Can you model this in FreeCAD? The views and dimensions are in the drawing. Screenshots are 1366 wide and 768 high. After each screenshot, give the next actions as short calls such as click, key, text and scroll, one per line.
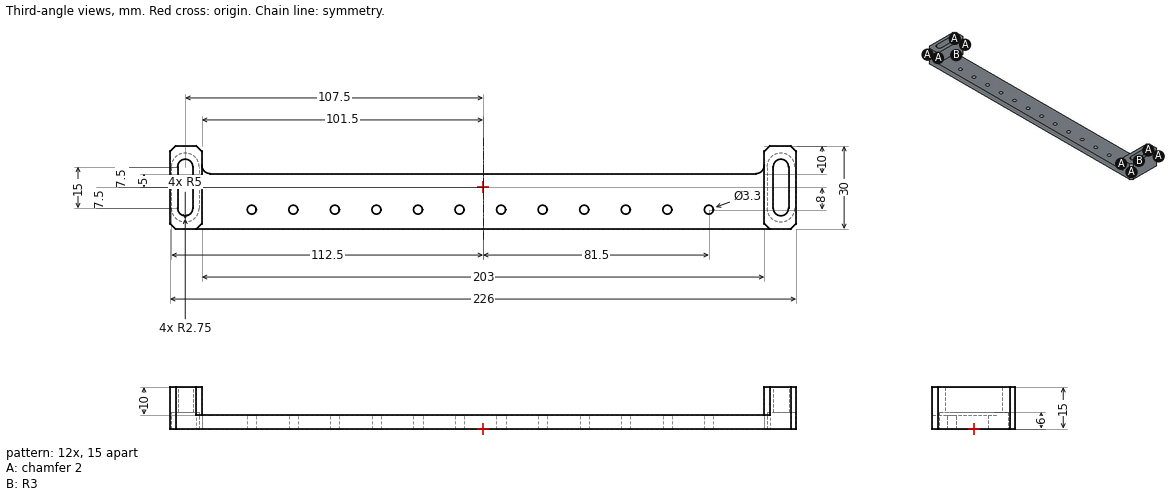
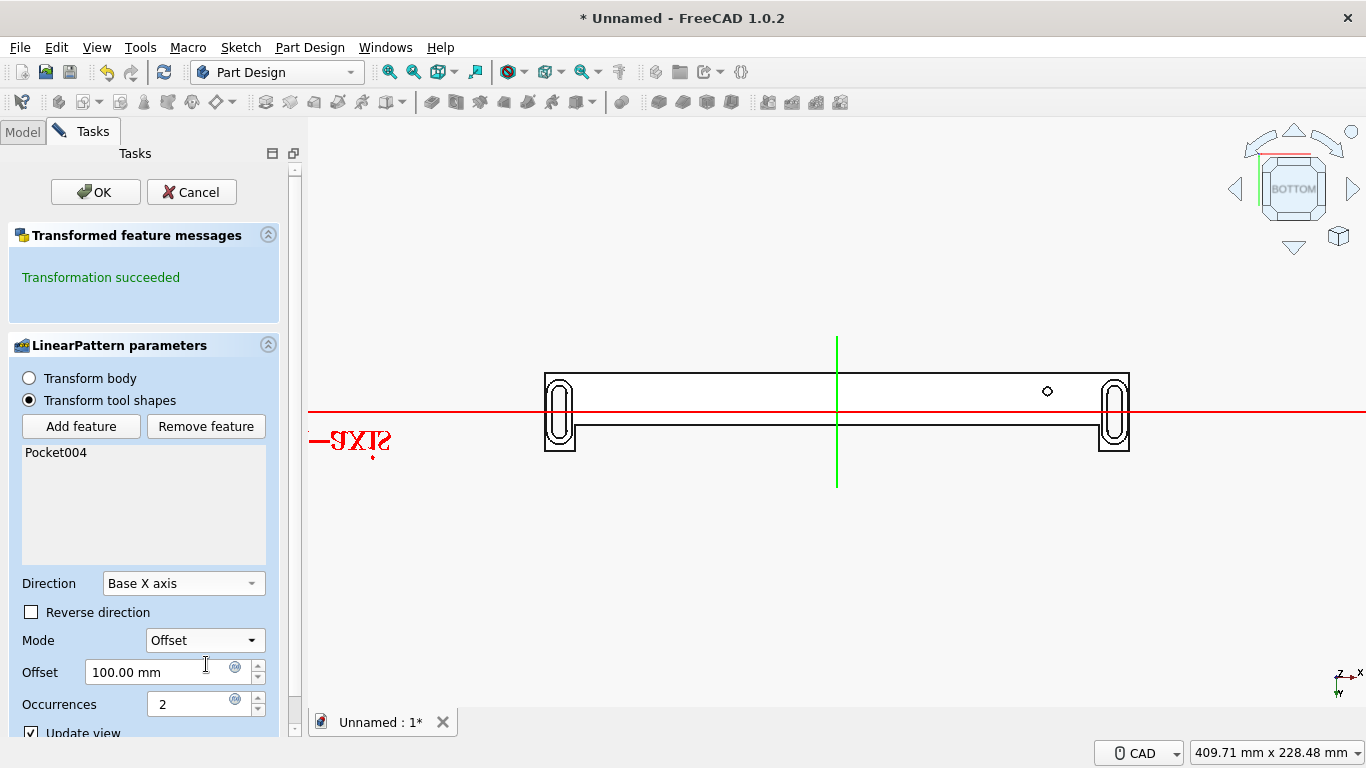
triple_click(168, 672)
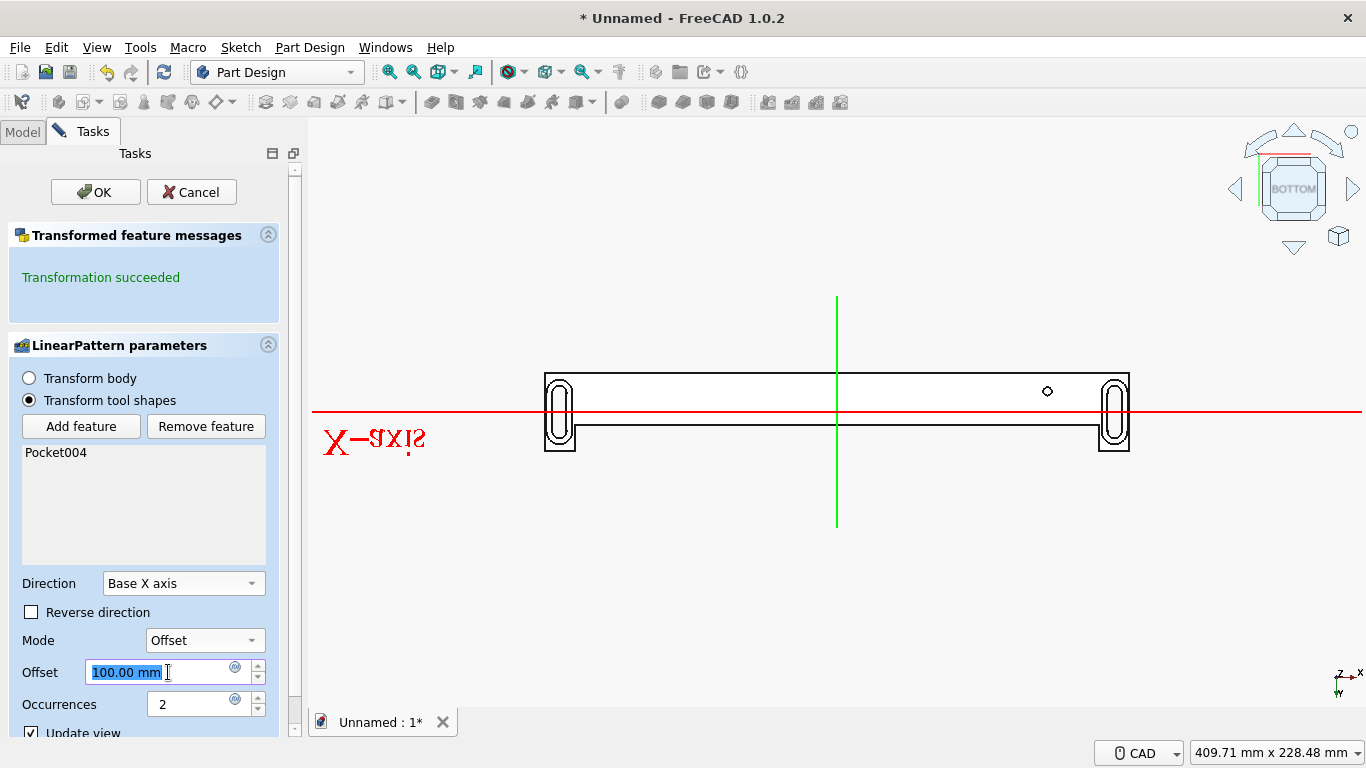
text(15)
key(Tab)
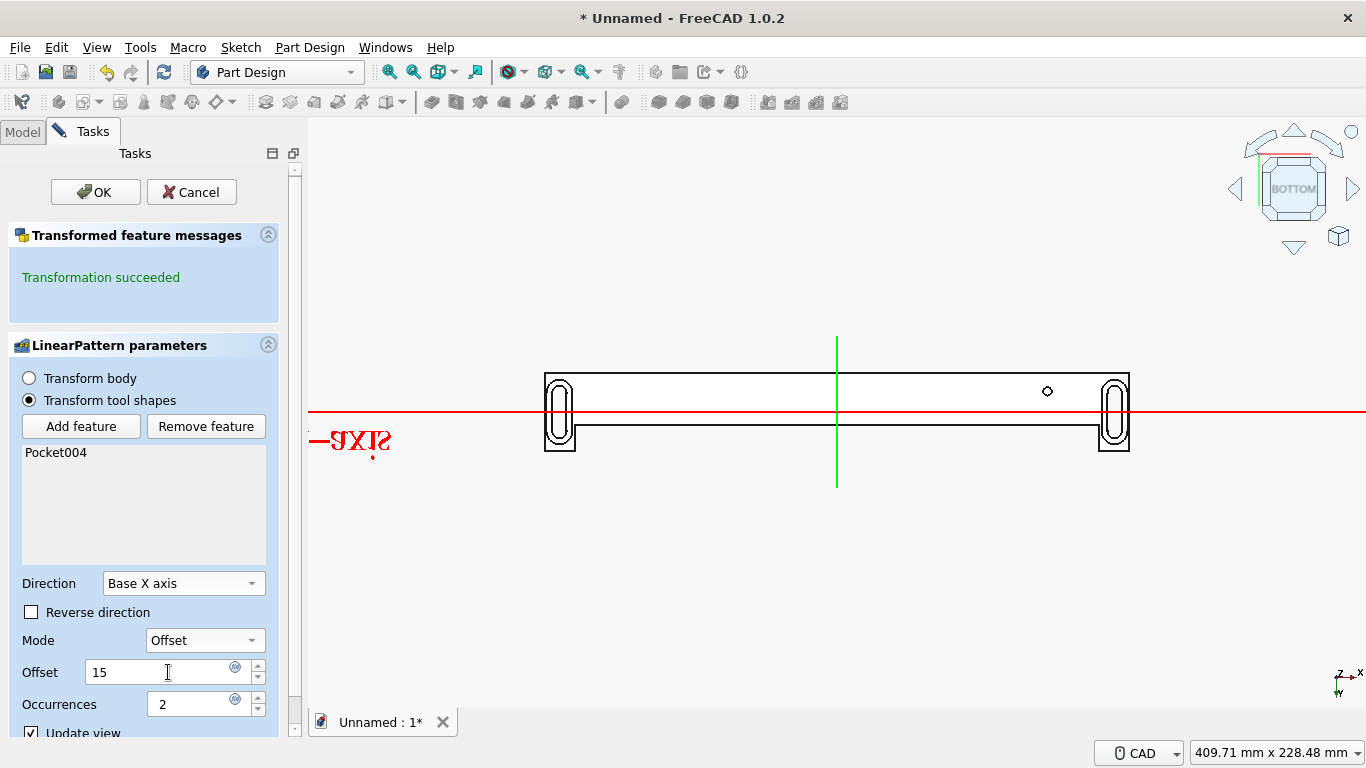
triple_click(198, 704)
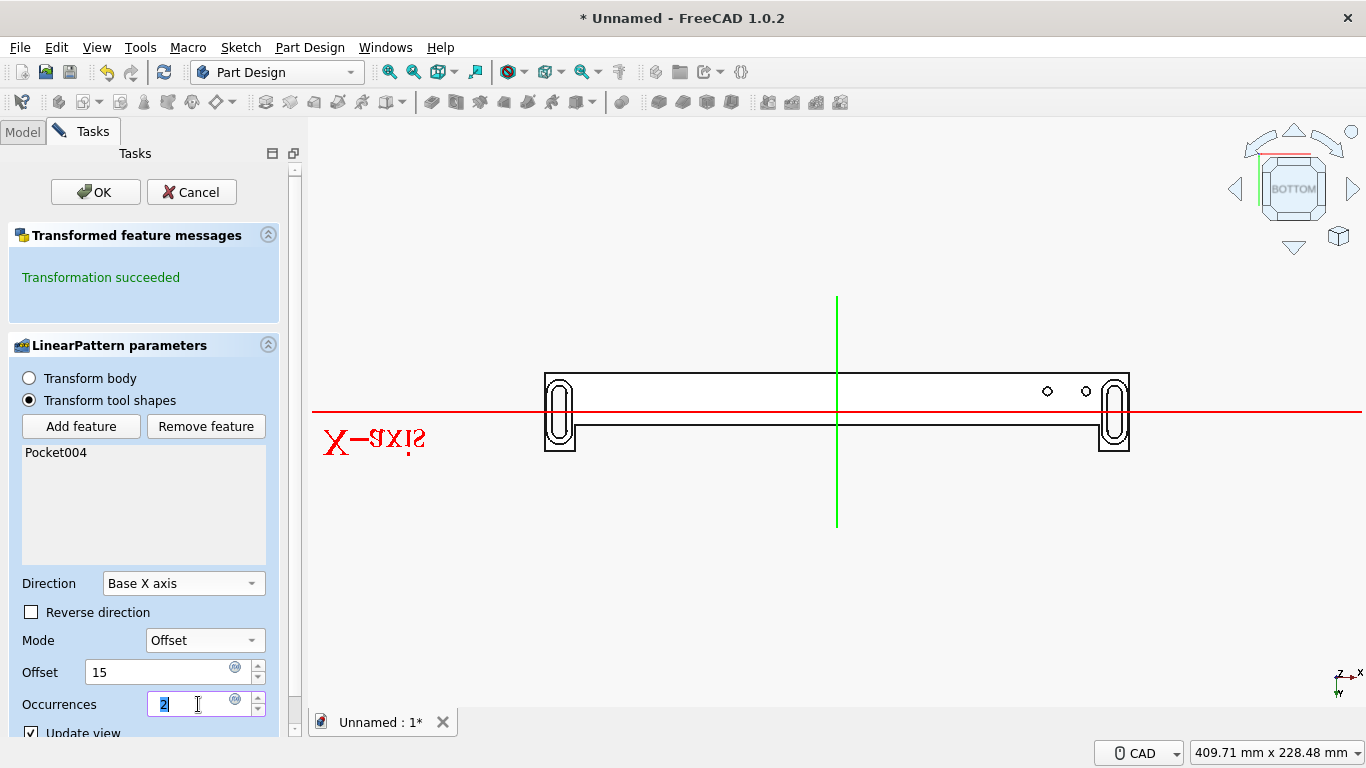
text(12)
key(Tab)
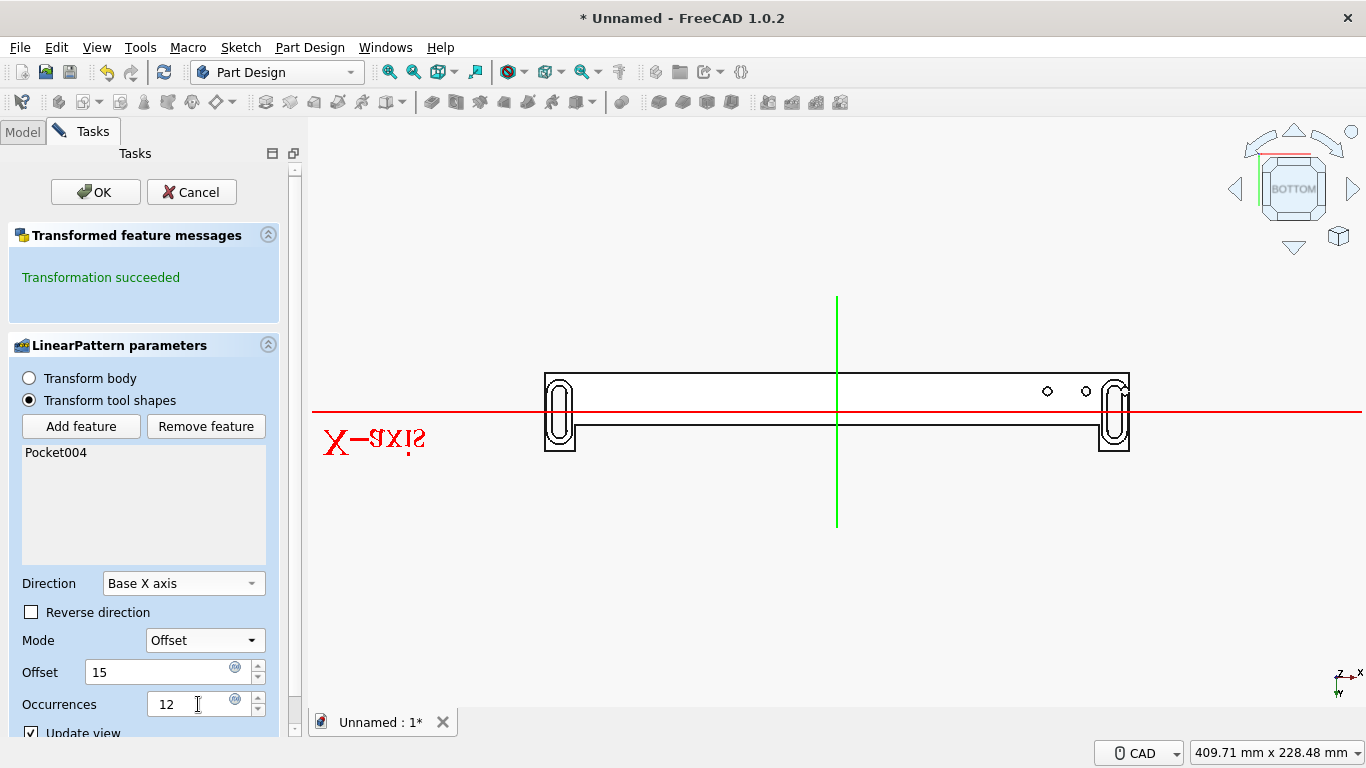
click(30, 612)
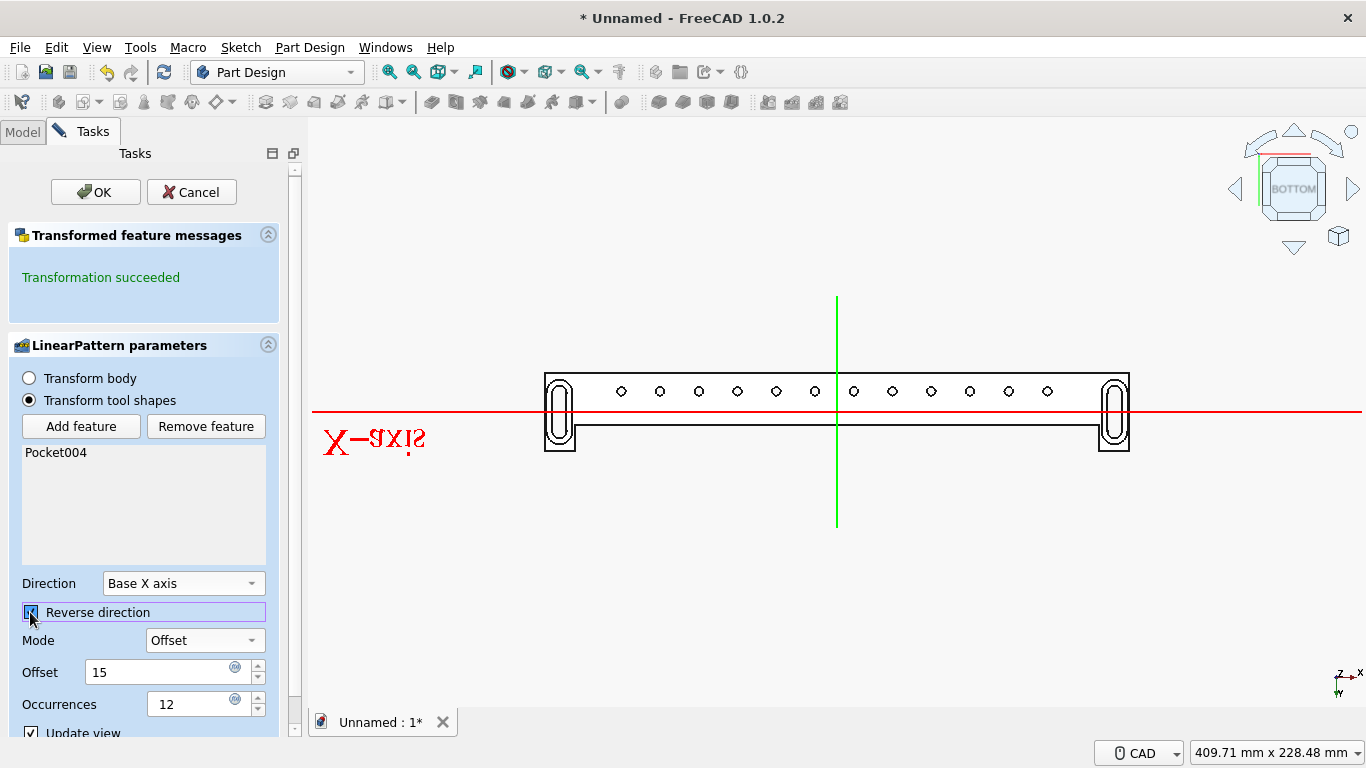
click(96, 192)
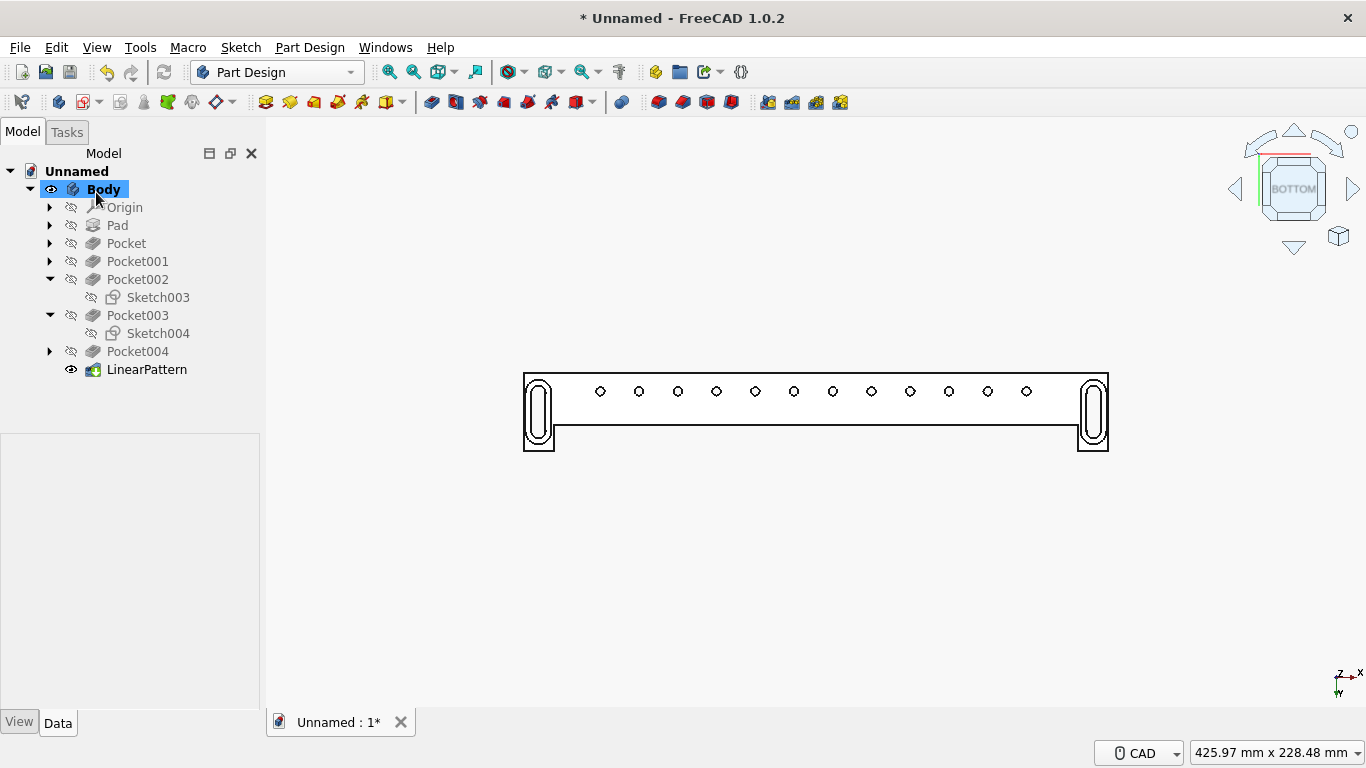
key(0)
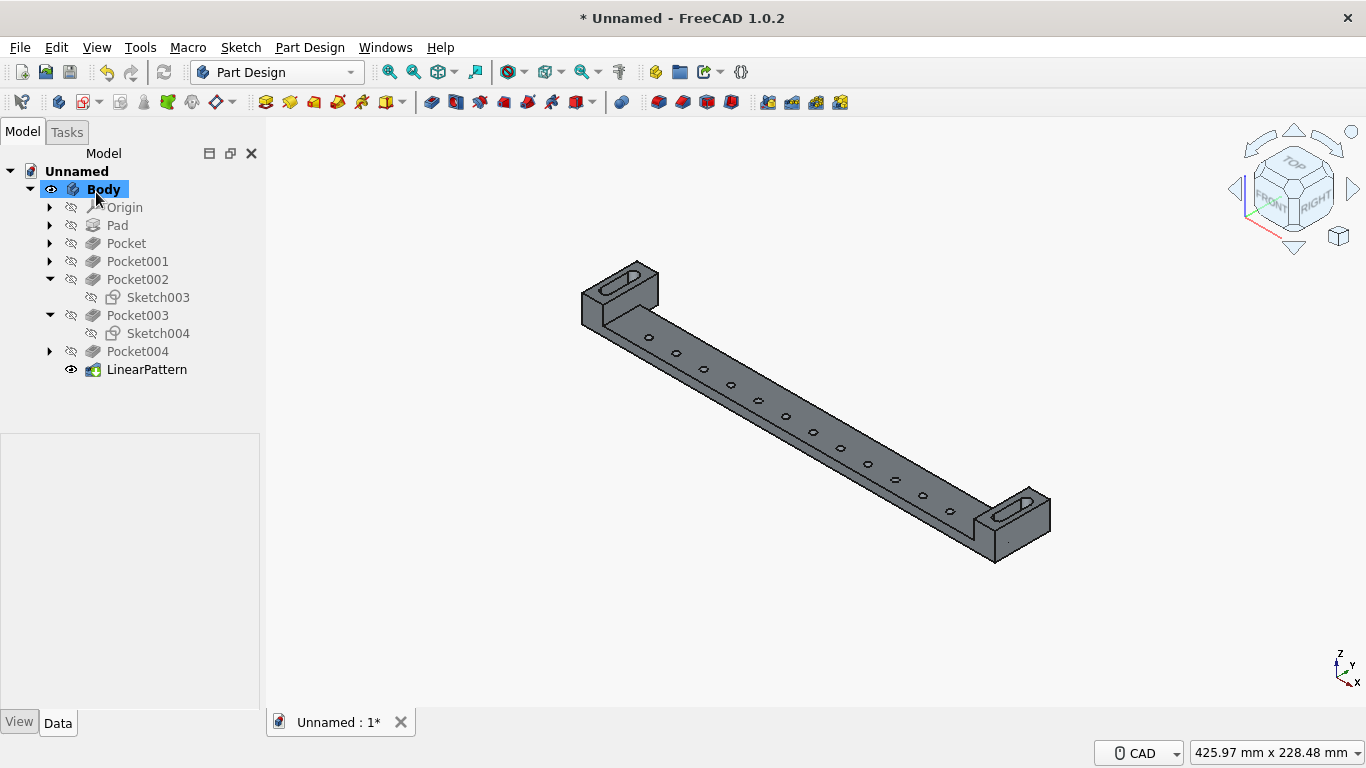
click(603, 315)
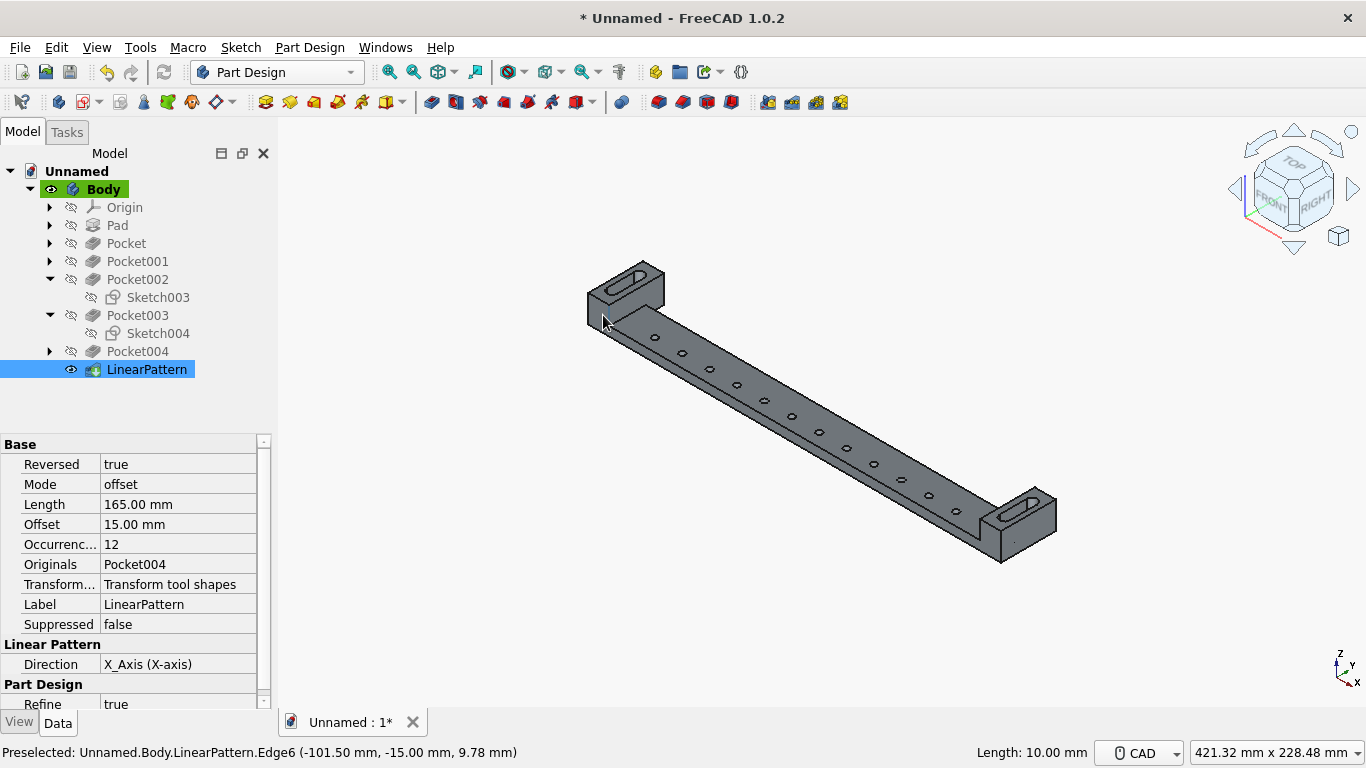
click(1001, 546, ctrl)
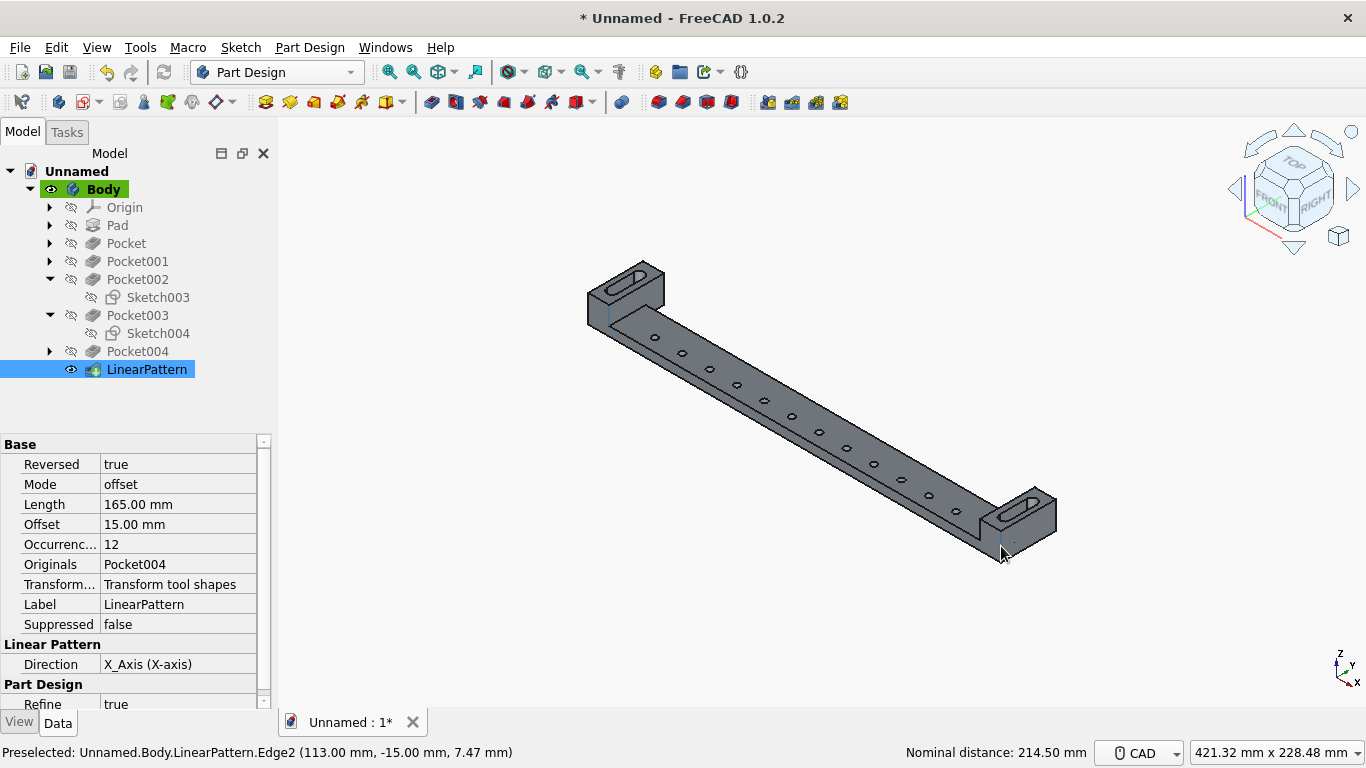
key(2)